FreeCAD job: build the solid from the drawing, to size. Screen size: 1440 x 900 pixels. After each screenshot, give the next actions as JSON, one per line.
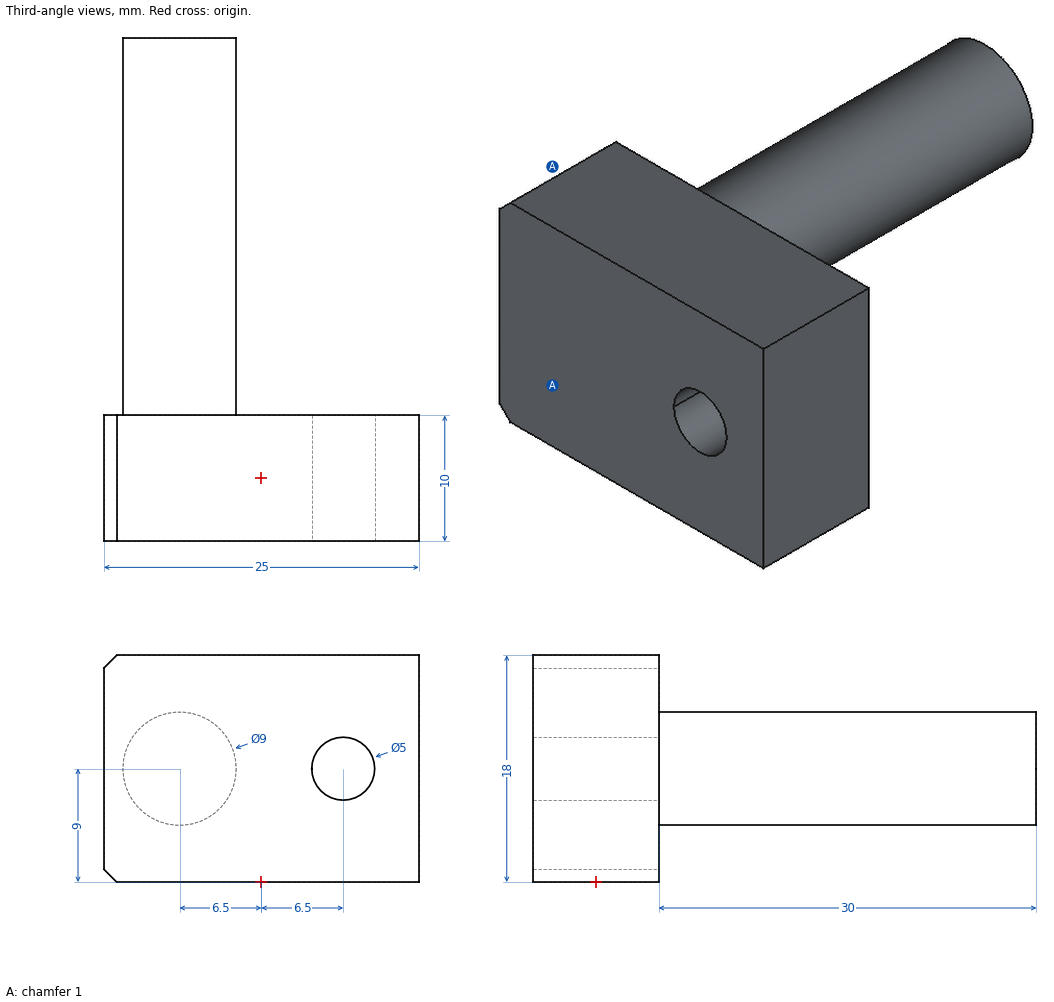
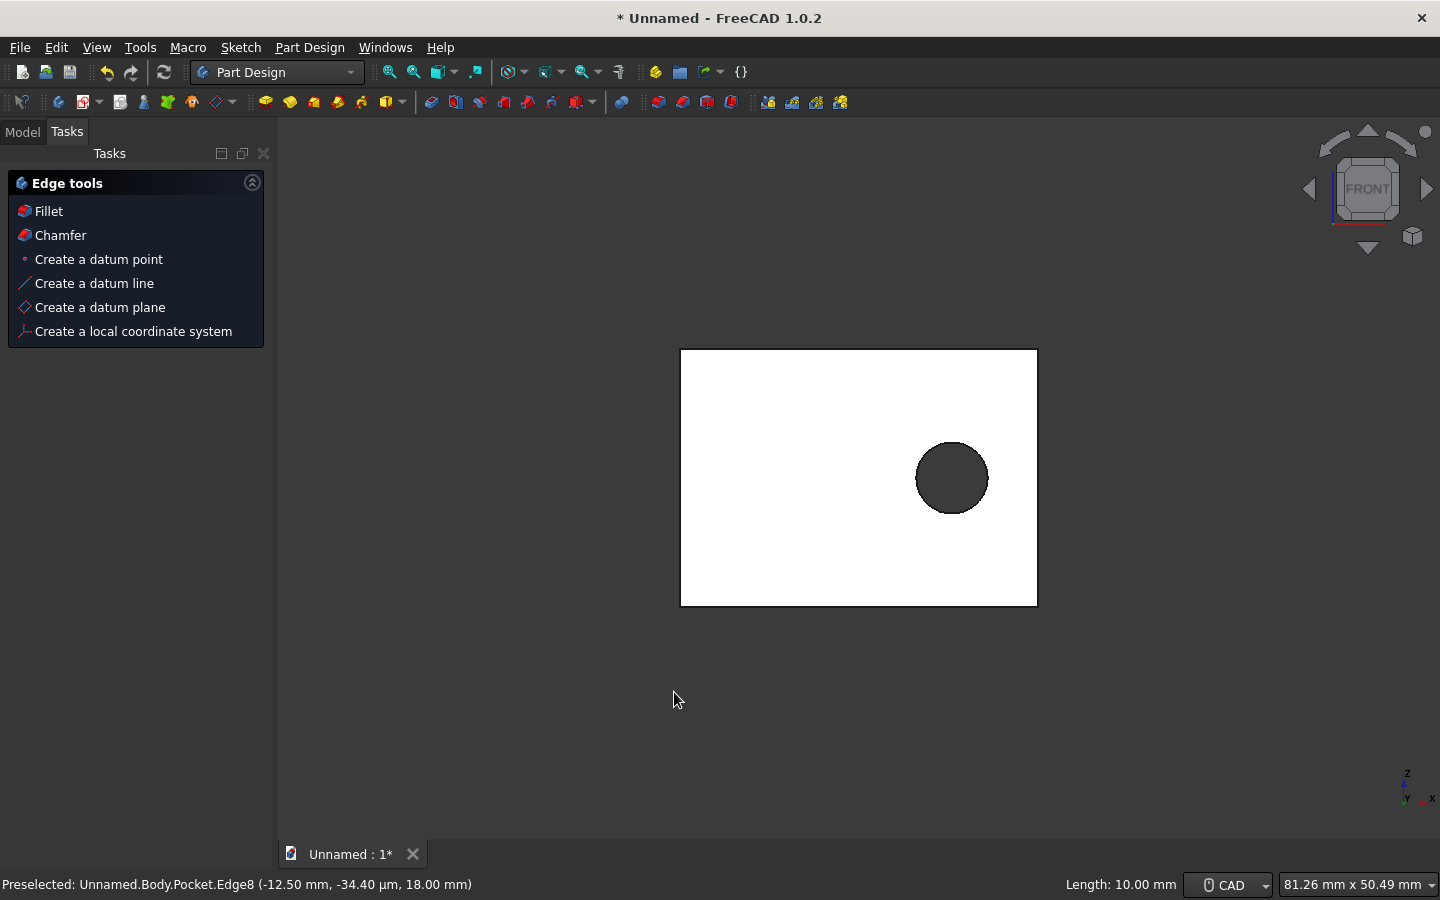
{"action": "key", "text": "3"}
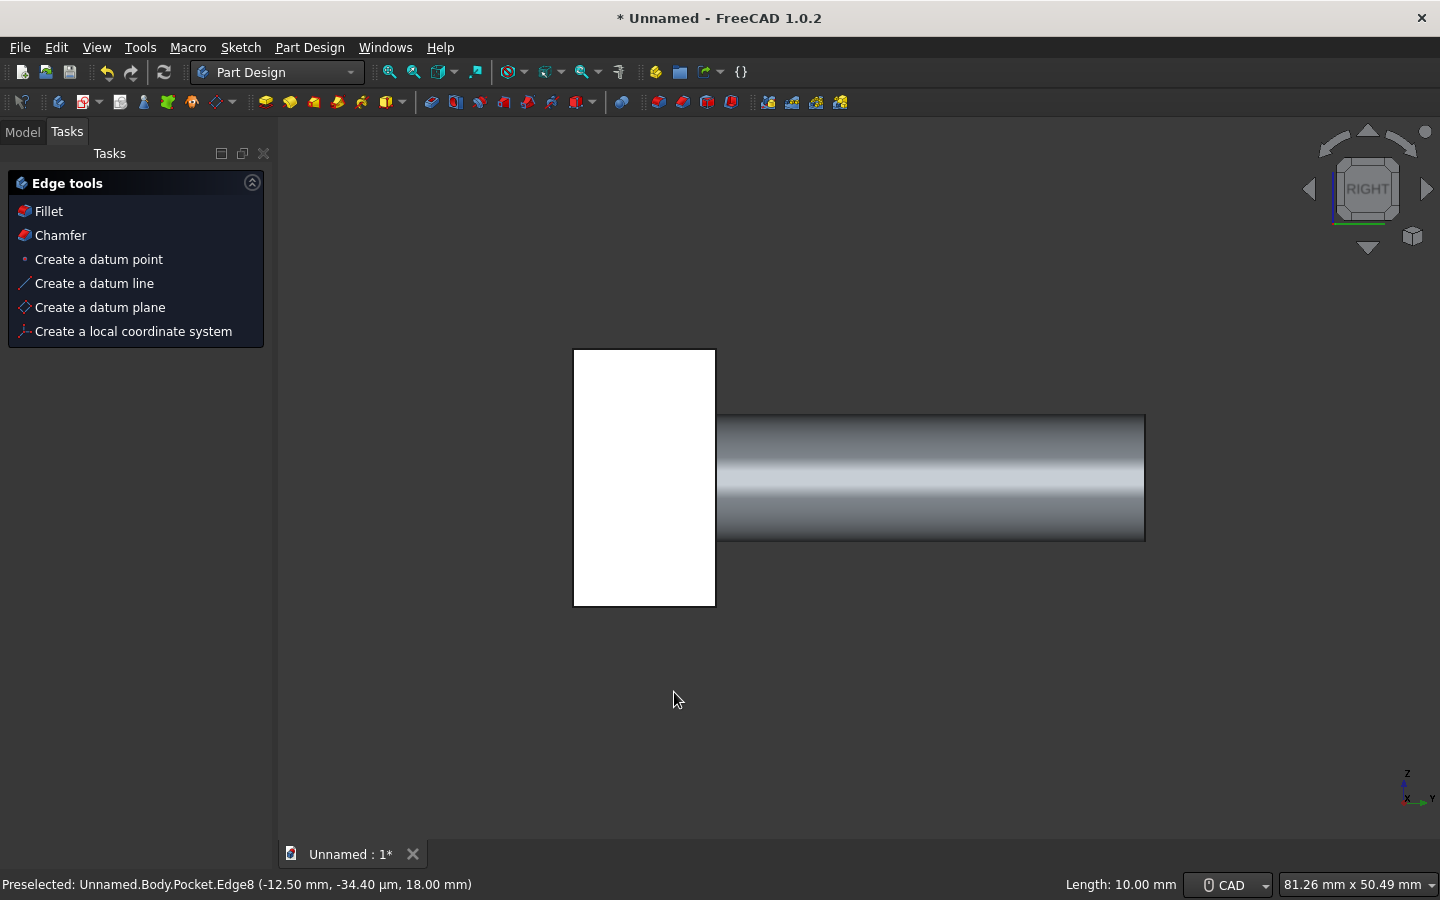
{"action": "key", "text": "5"}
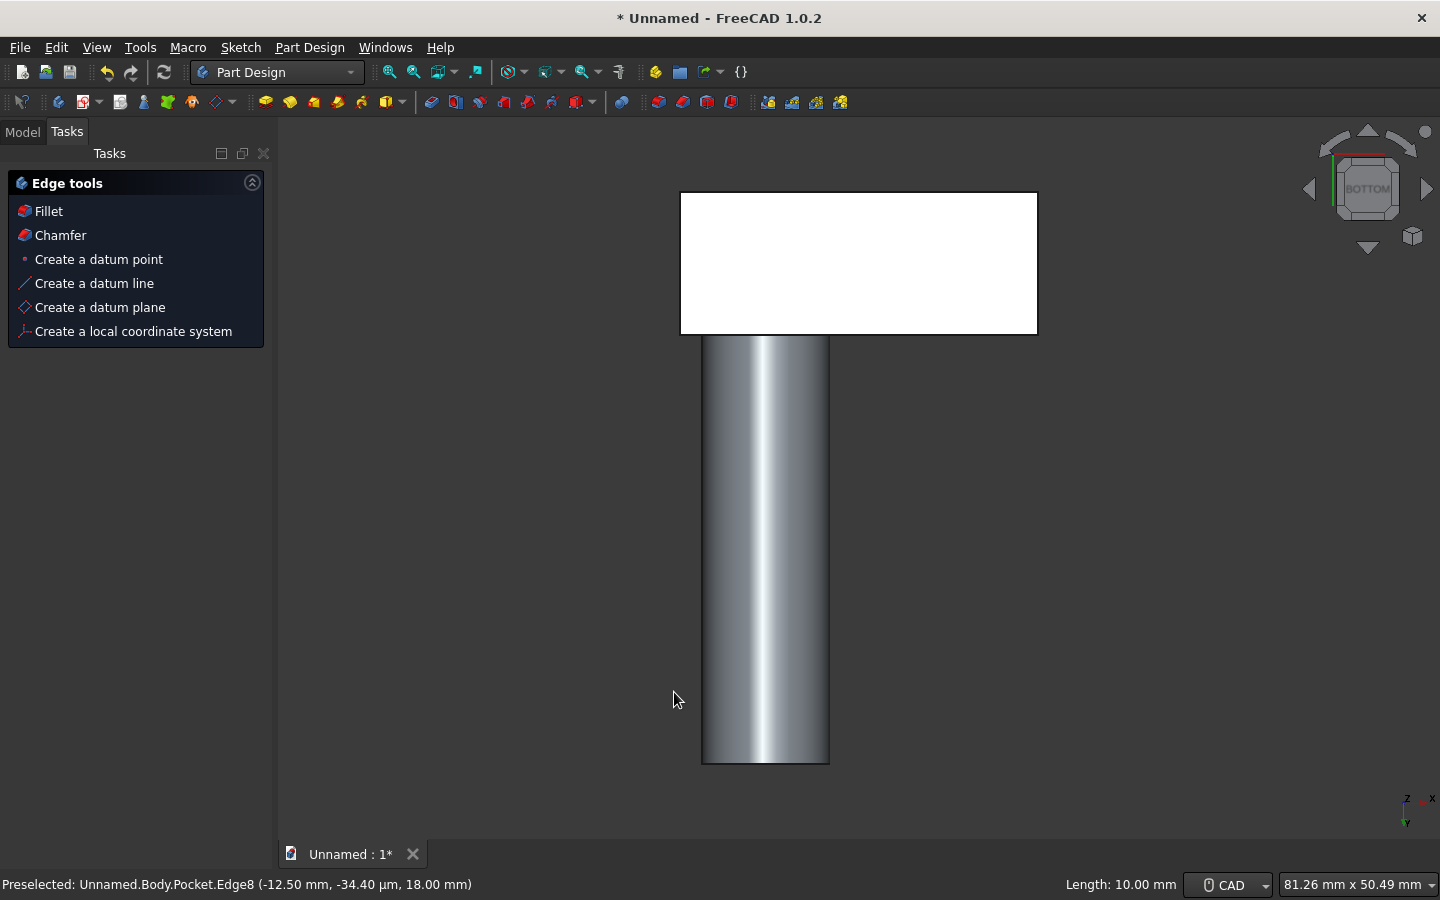
{"action": "left_click", "coordinate": [680, 262], "text": "ctrl"}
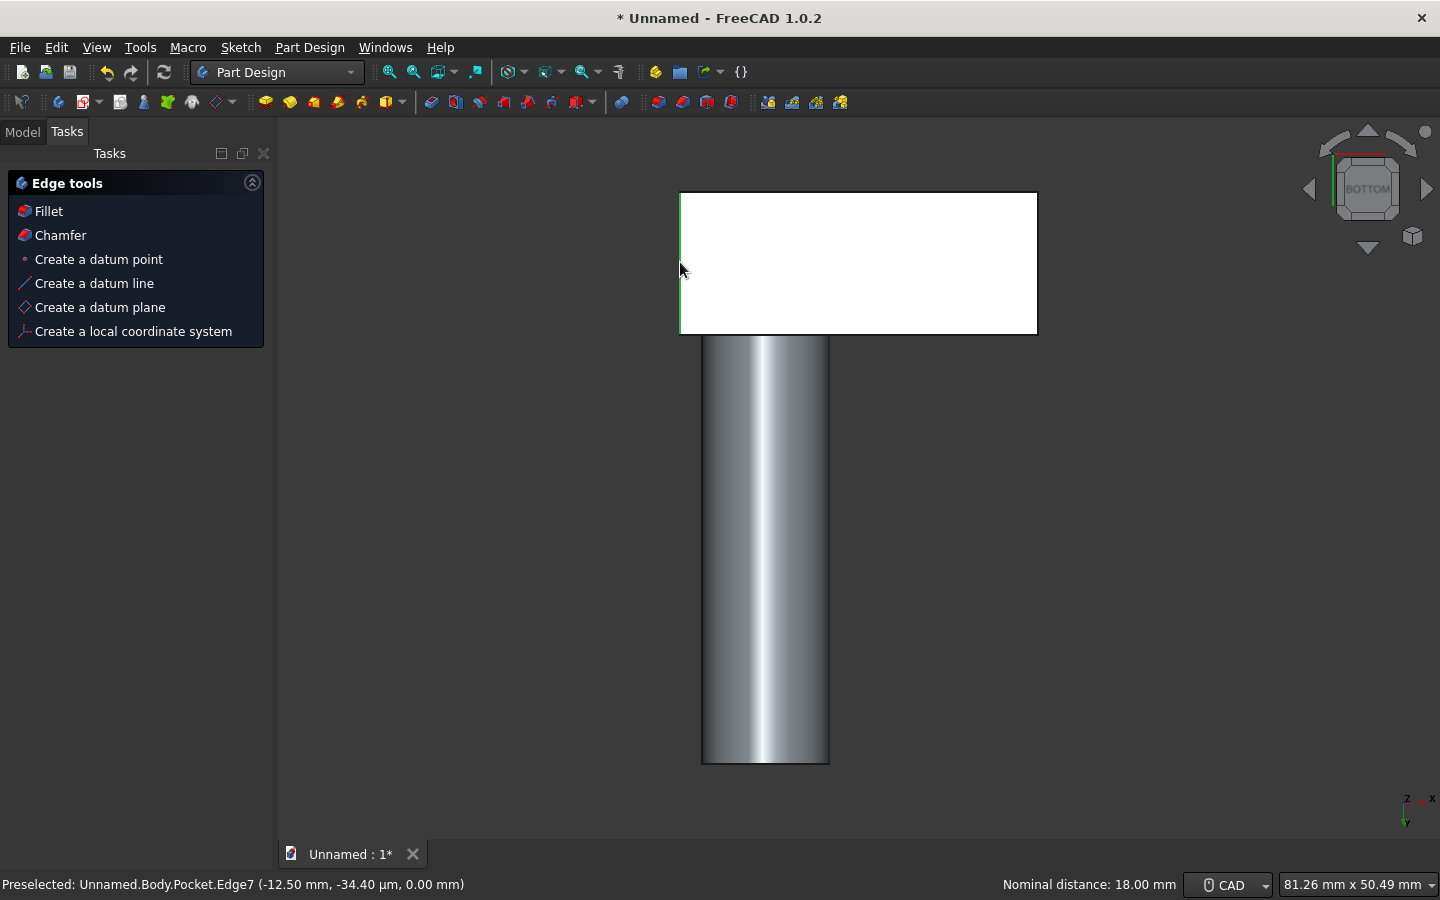
{"action": "left_click", "coordinate": [684, 102]}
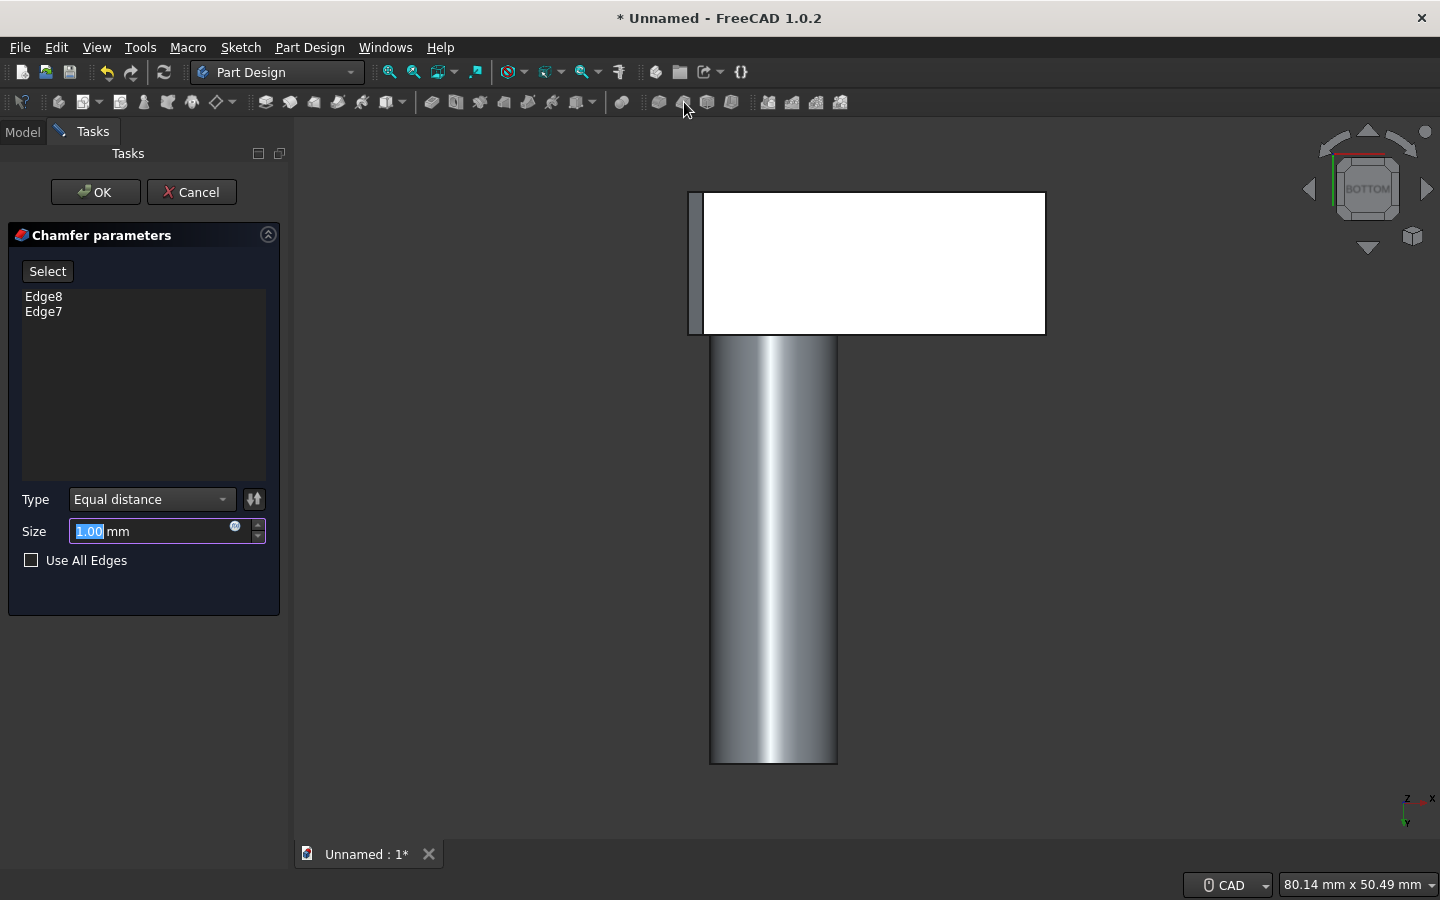
{"action": "type", "text": "1"}
{"action": "key", "text": "Tab"}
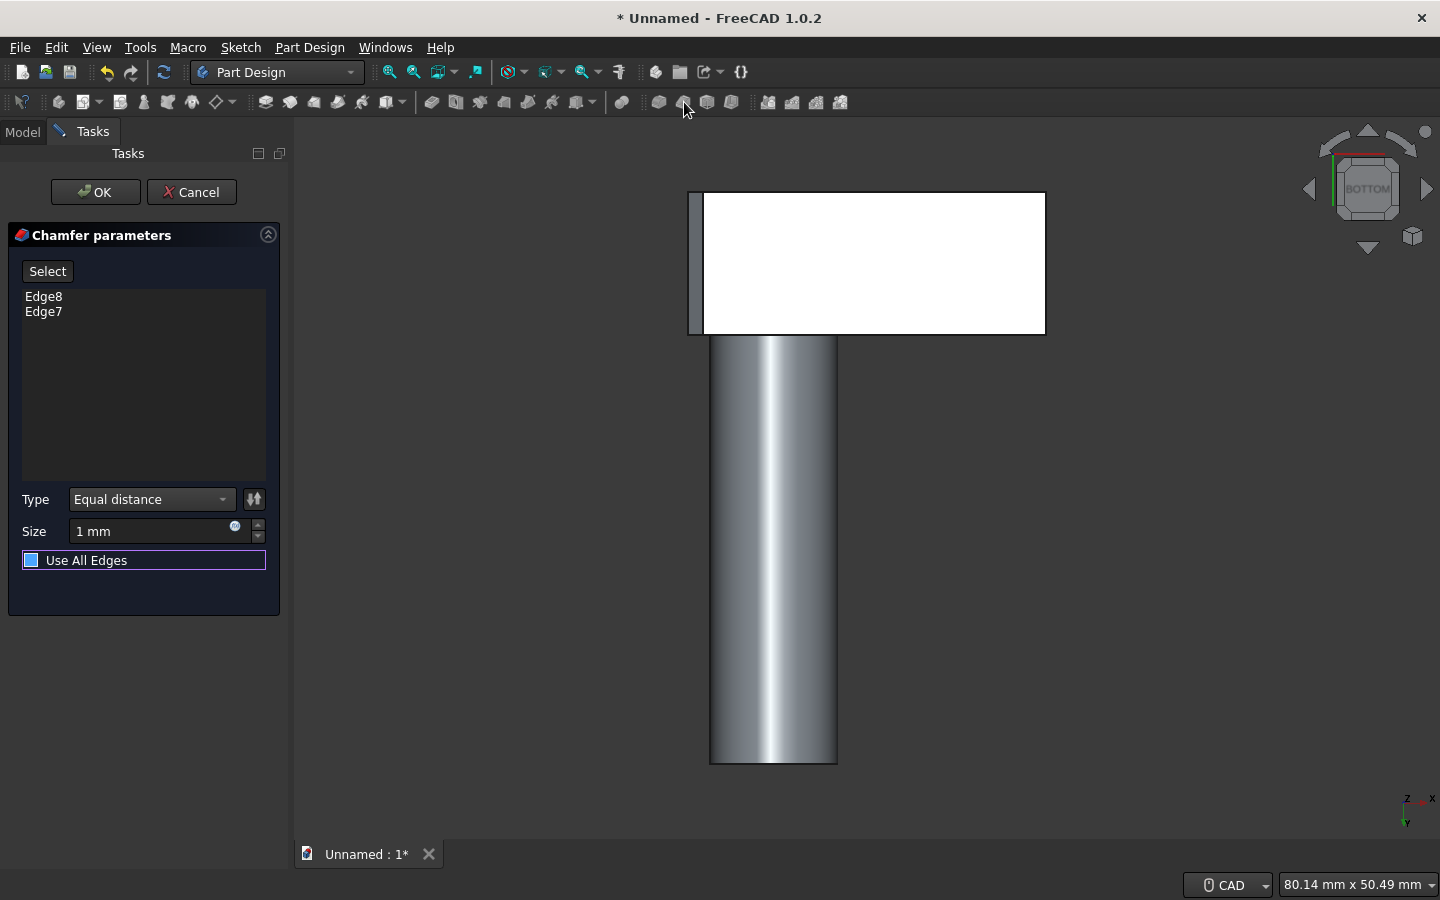
{"action": "left_click", "coordinate": [96, 192]}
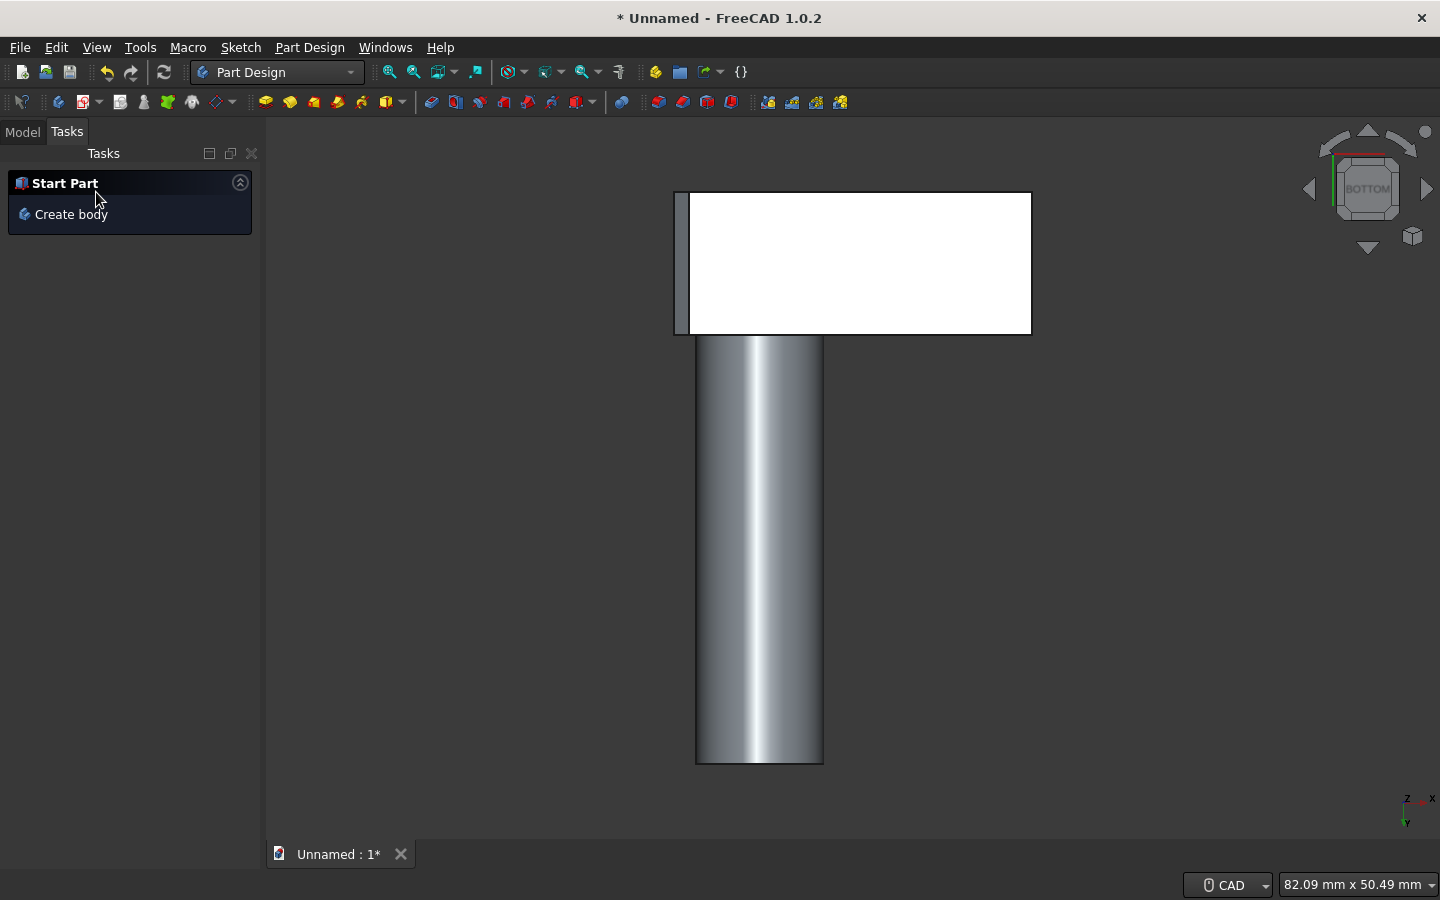
{"action": "key", "text": "0"}